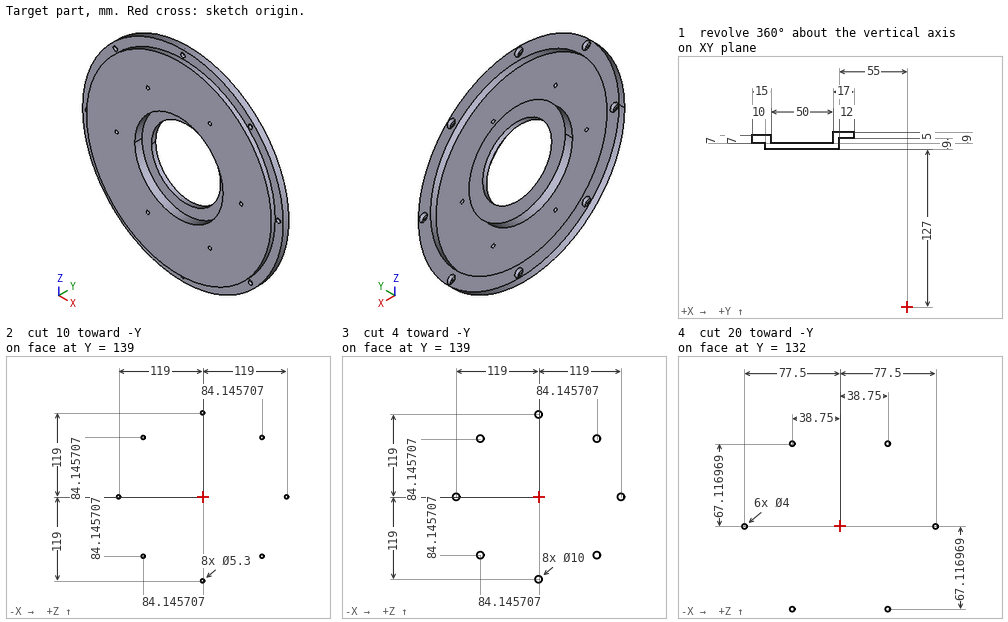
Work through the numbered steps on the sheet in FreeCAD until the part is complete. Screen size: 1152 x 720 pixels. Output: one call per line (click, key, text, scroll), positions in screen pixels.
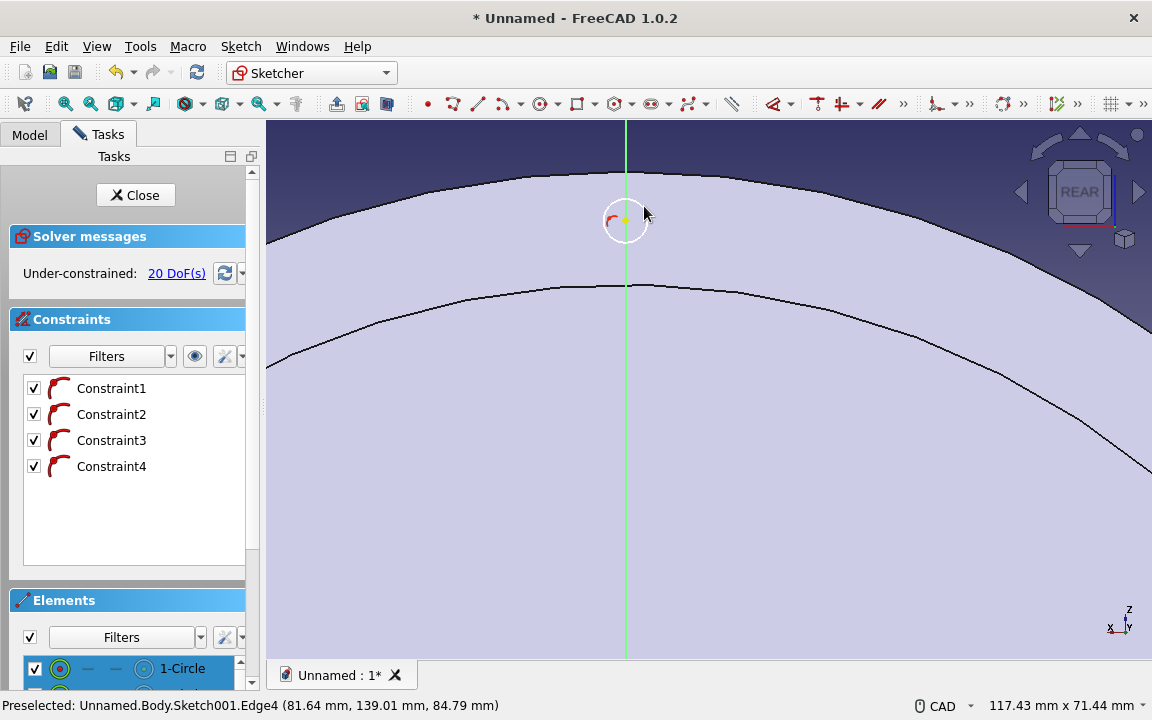
click(641, 205)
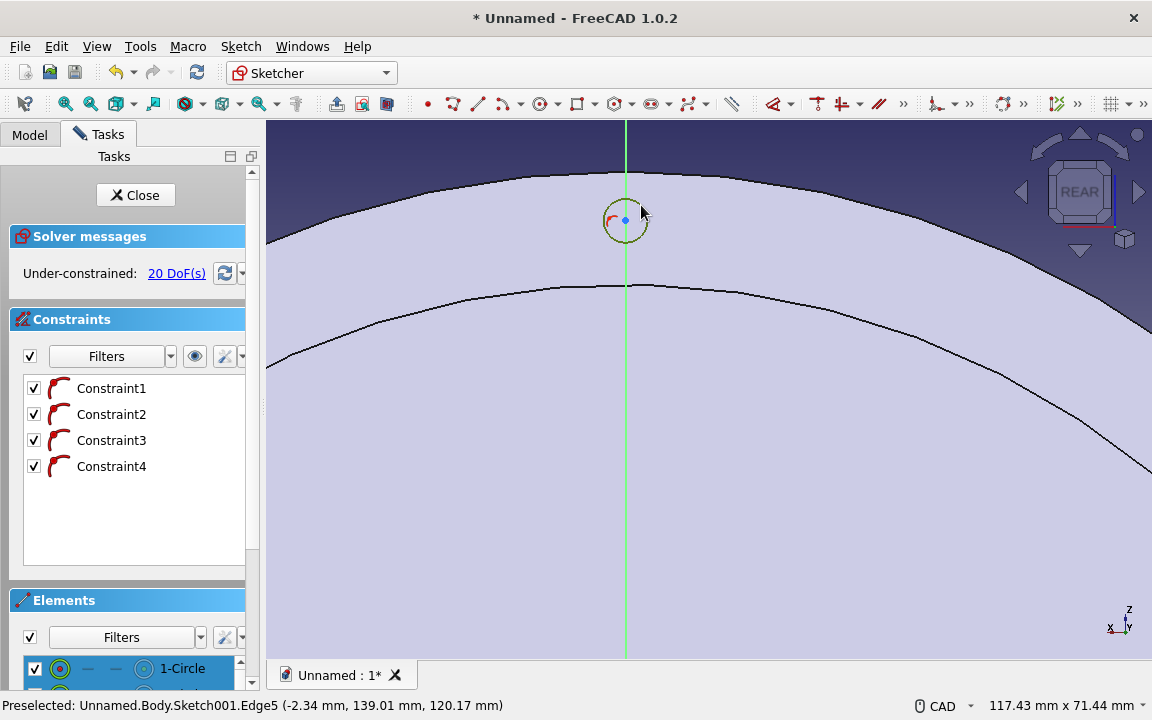
scroll(644, 206, down, 8)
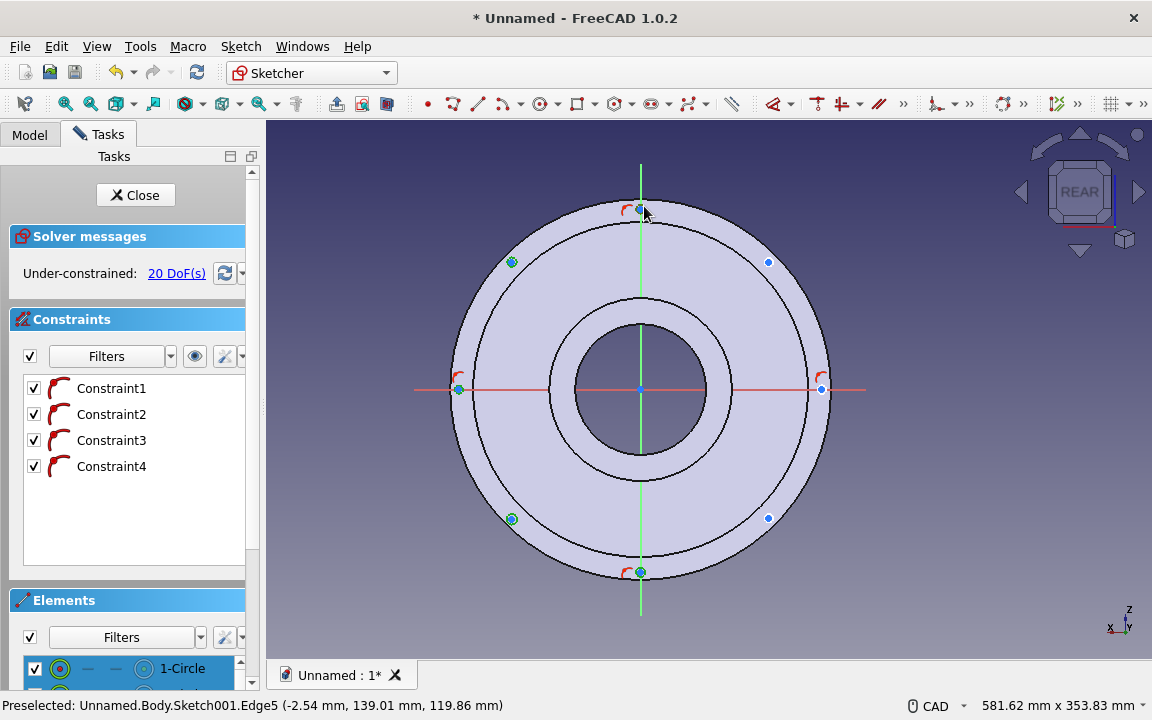
scroll(772, 259, up, 6)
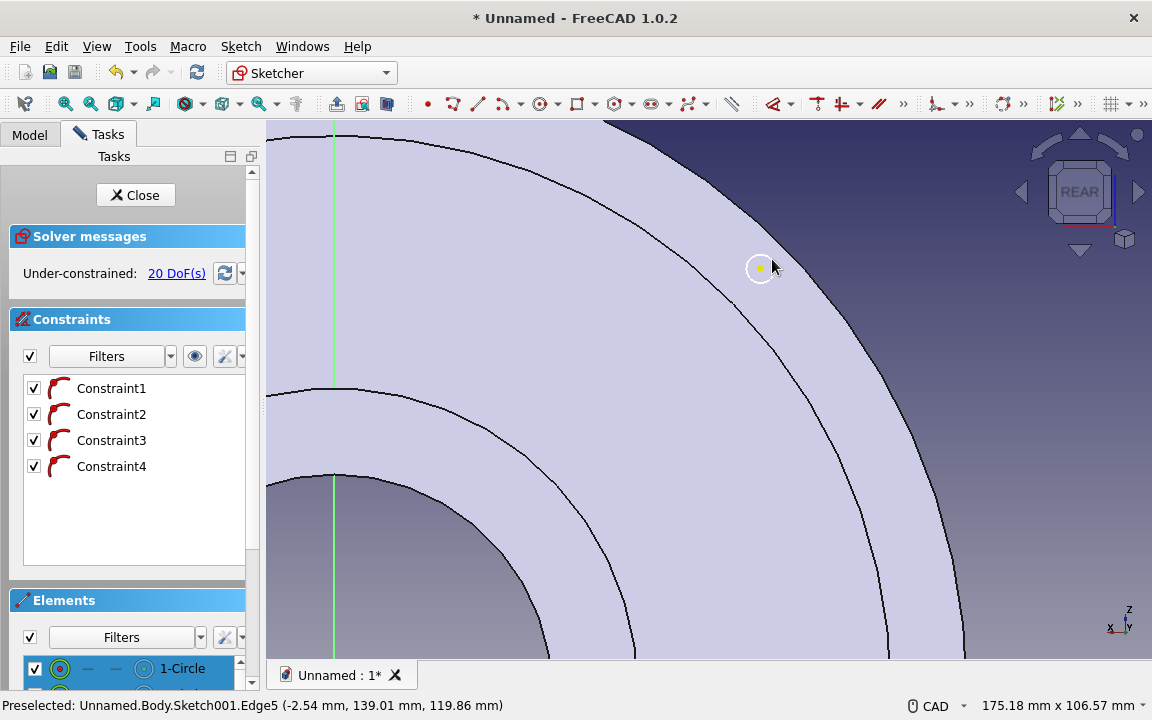
click(771, 259)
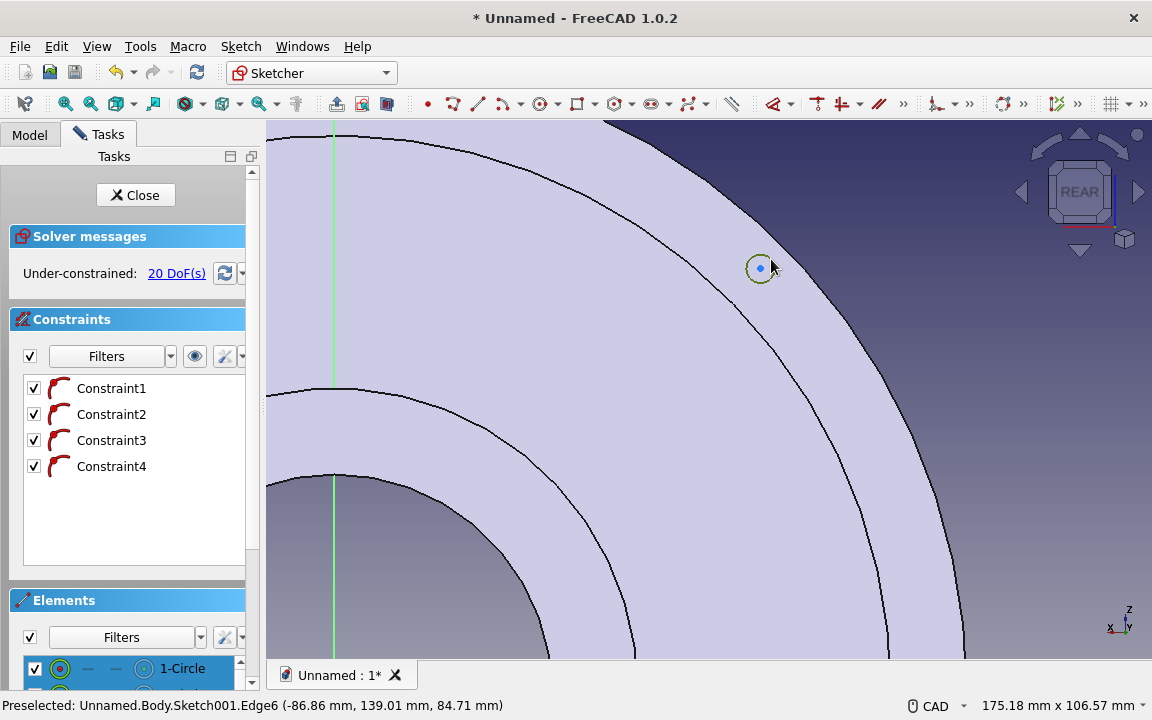
scroll(772, 259, down, 6)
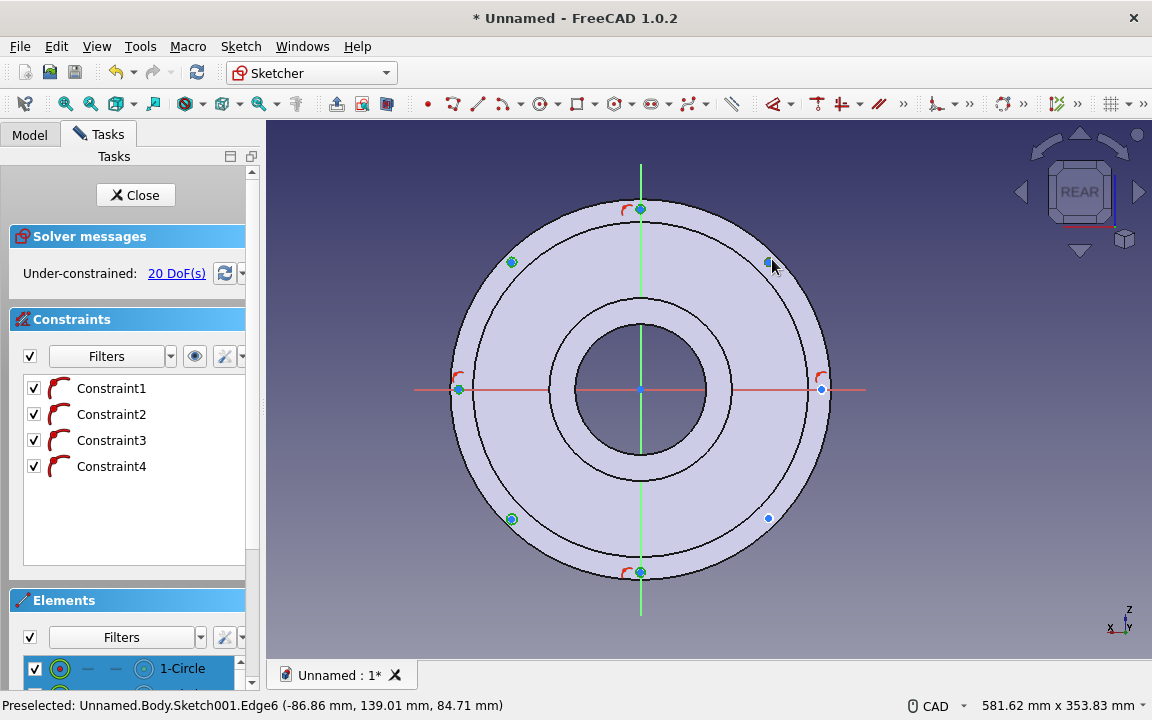
scroll(825, 387, up, 8)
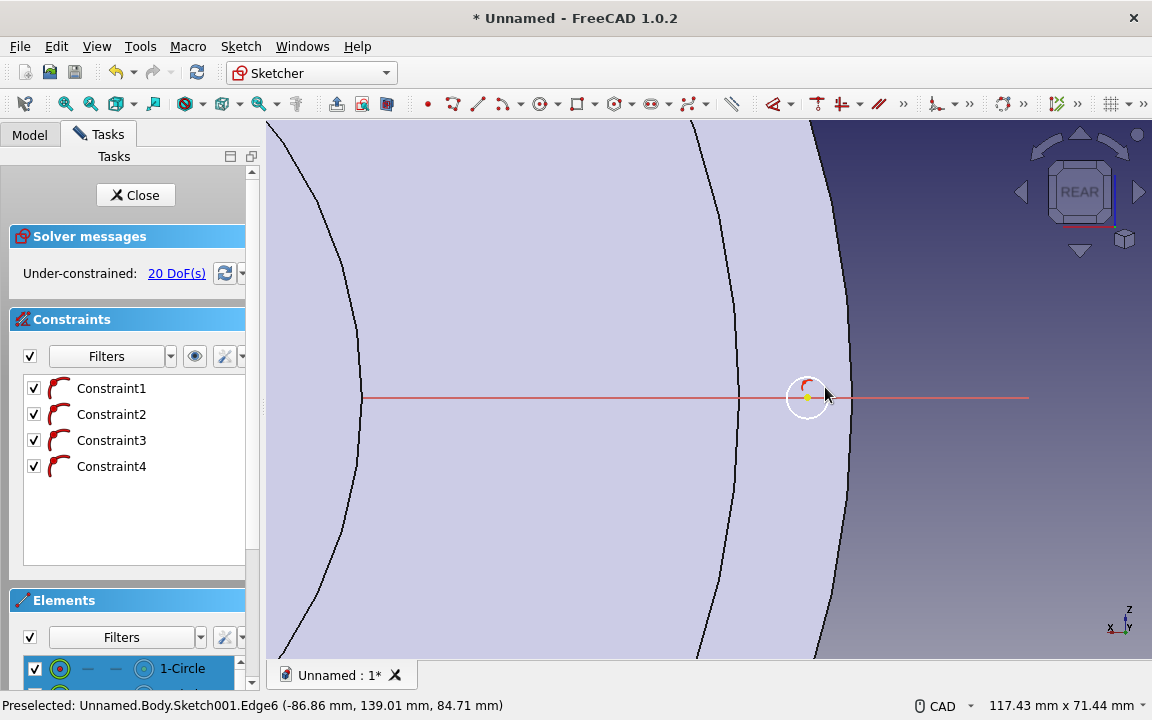
click(822, 383)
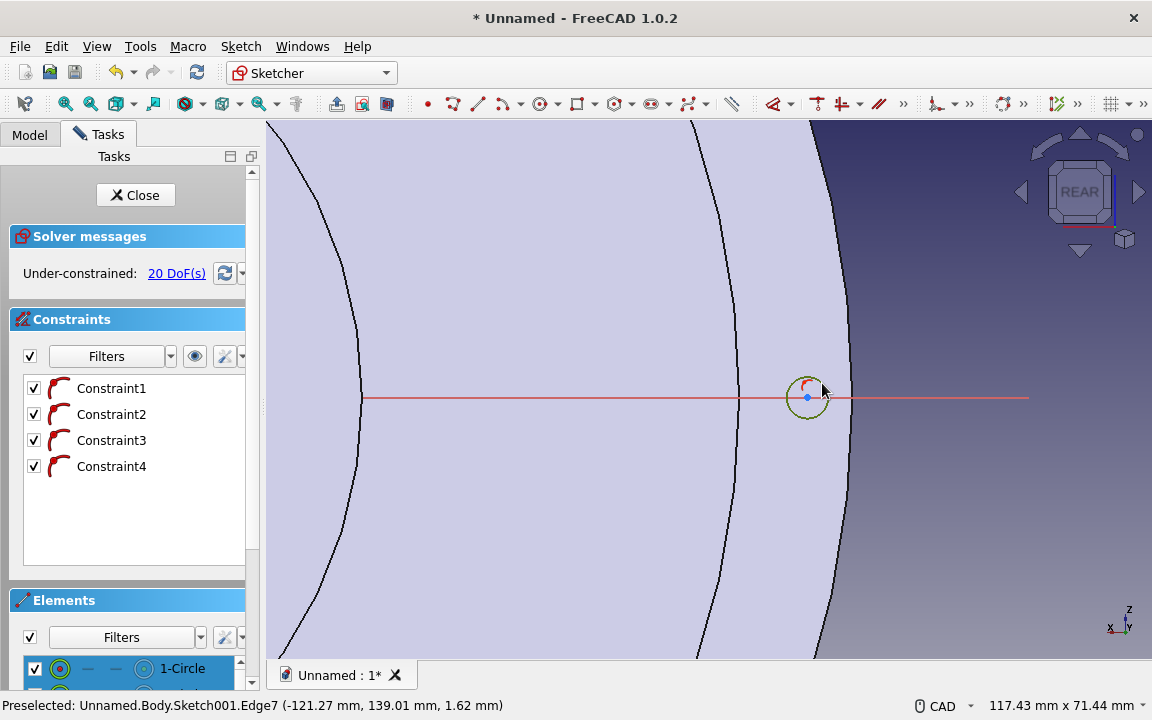
scroll(825, 387, down, 8)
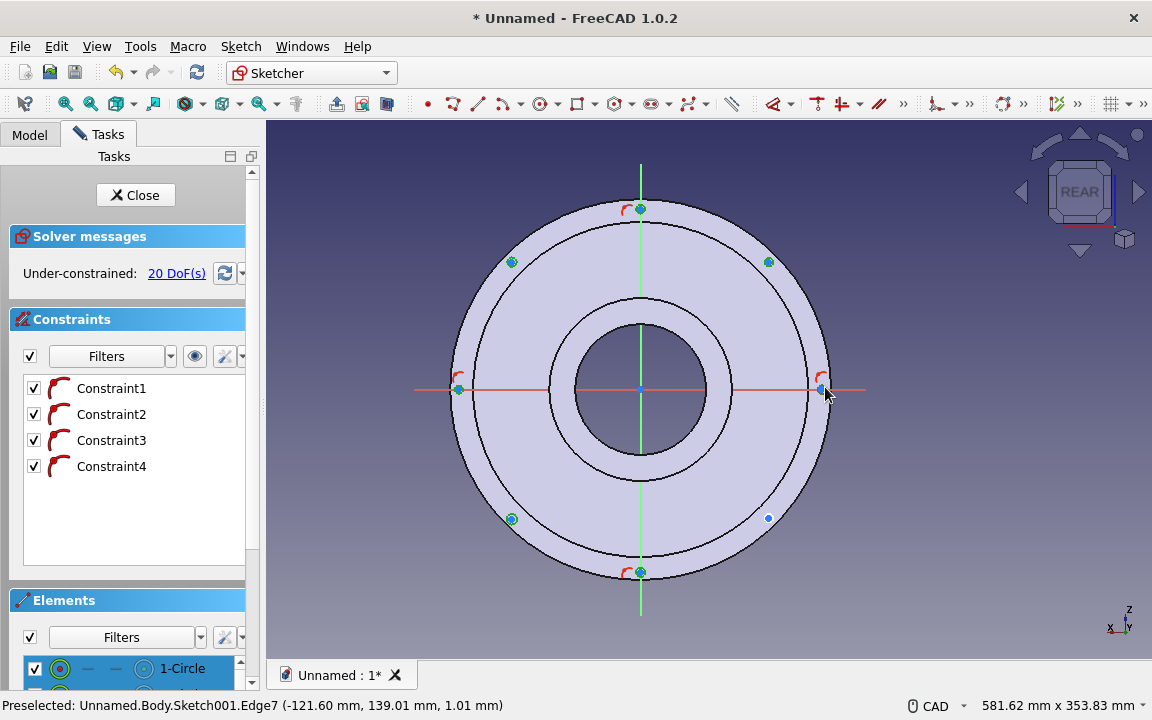
scroll(772, 515, up, 6)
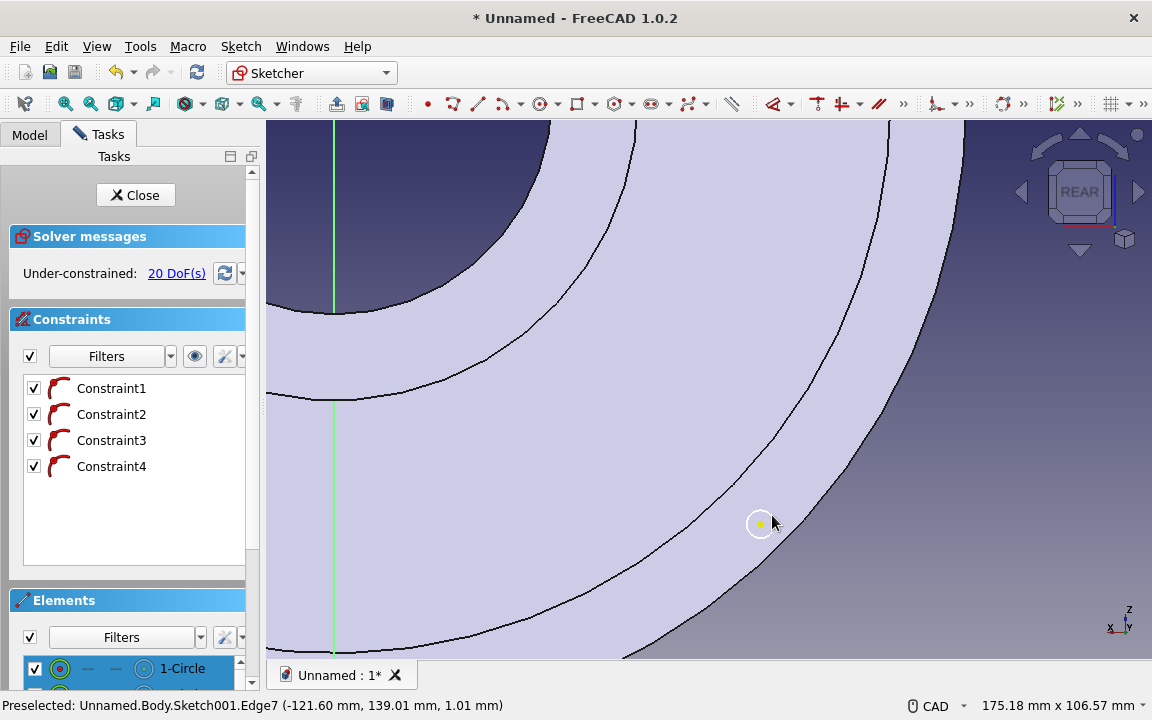
click(770, 514)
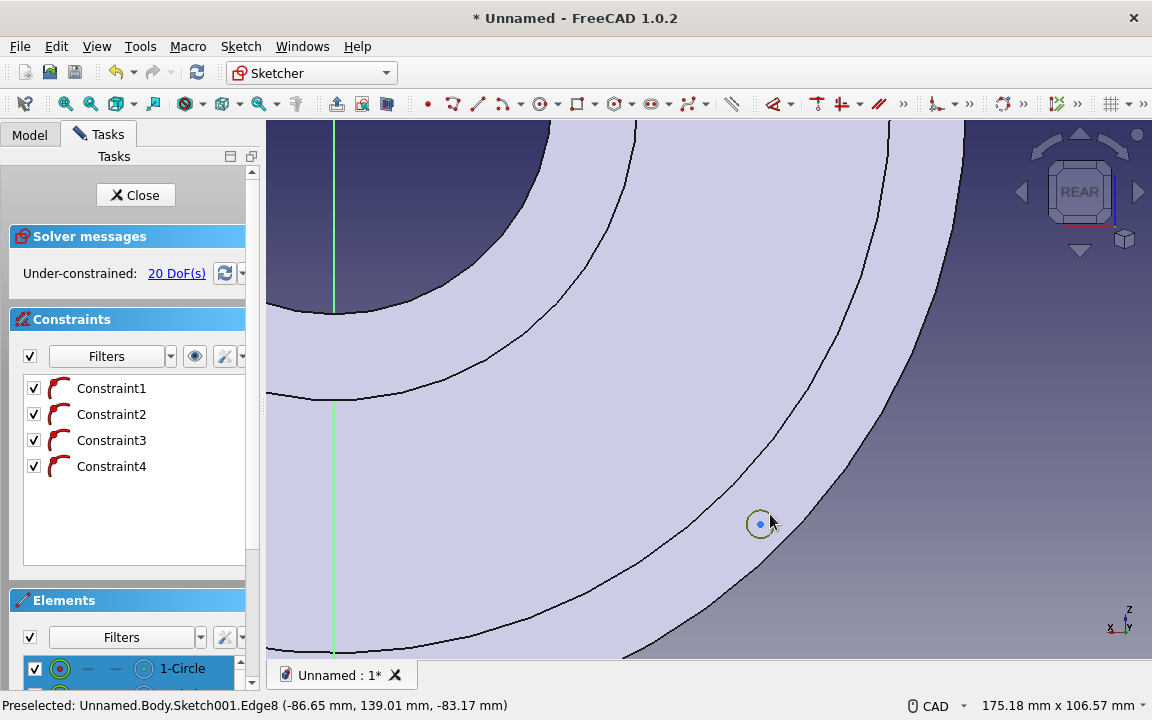
key(e)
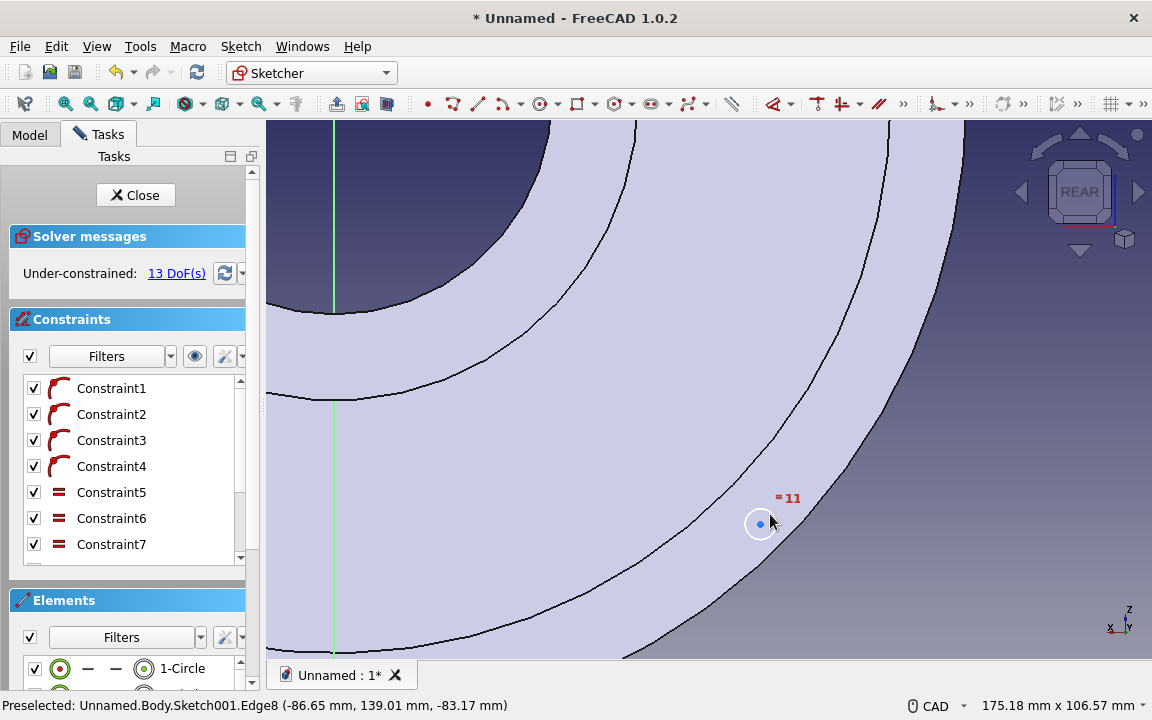
scroll(772, 516, down, 6)